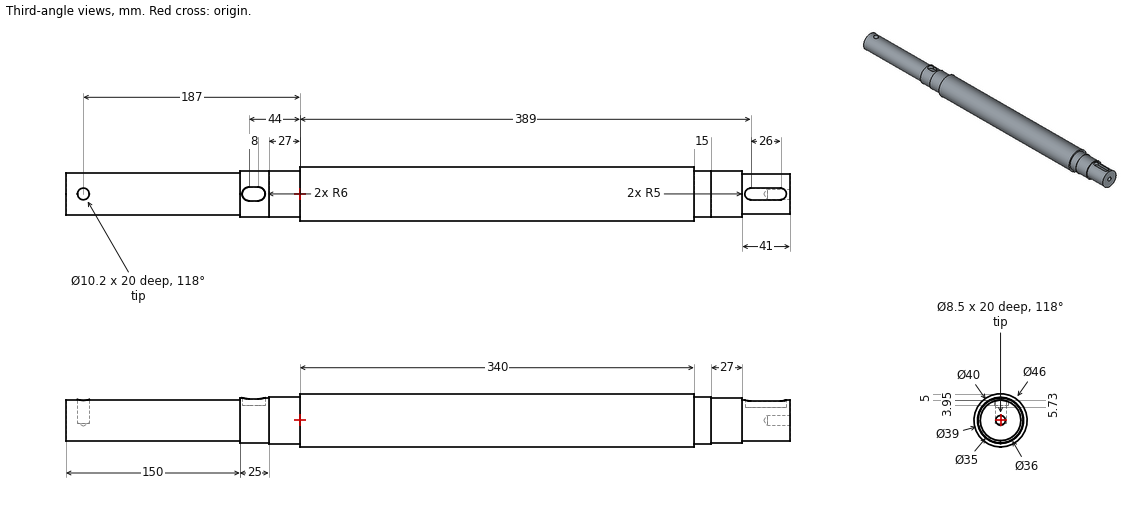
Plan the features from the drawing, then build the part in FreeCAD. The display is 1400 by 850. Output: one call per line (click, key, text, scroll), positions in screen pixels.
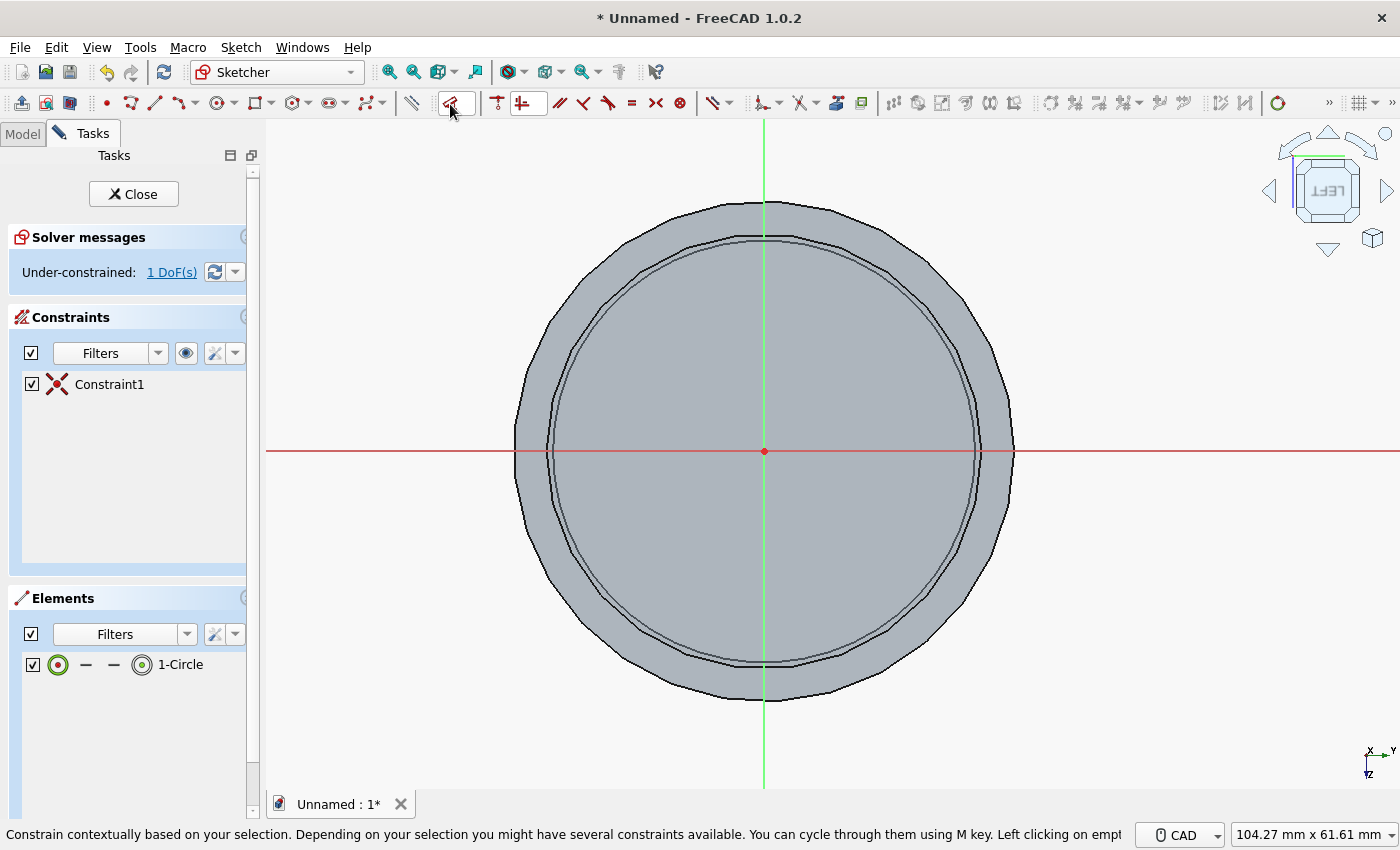
click(913, 302)
click(936, 279)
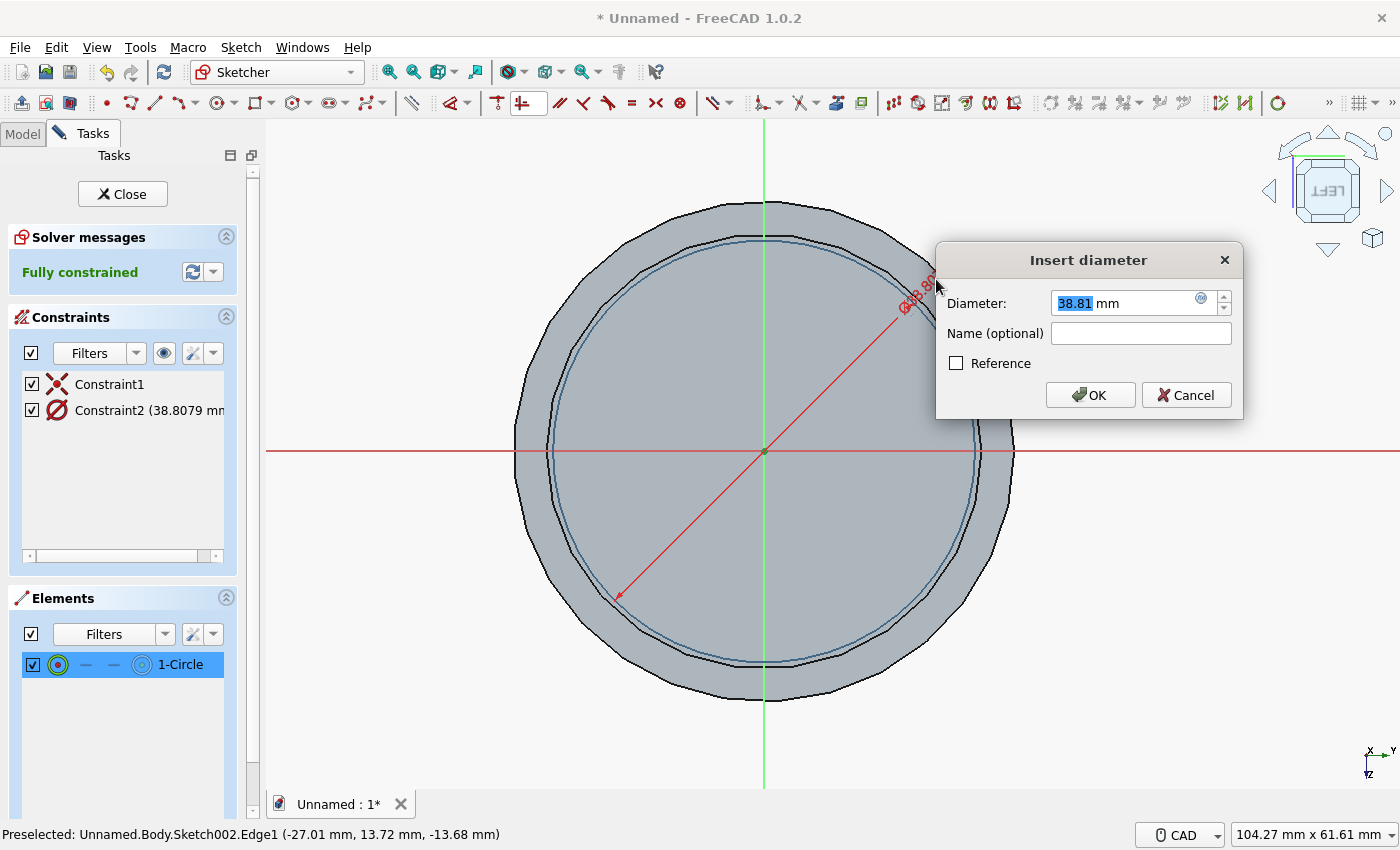
text(39)
key(Return)
key(Escape)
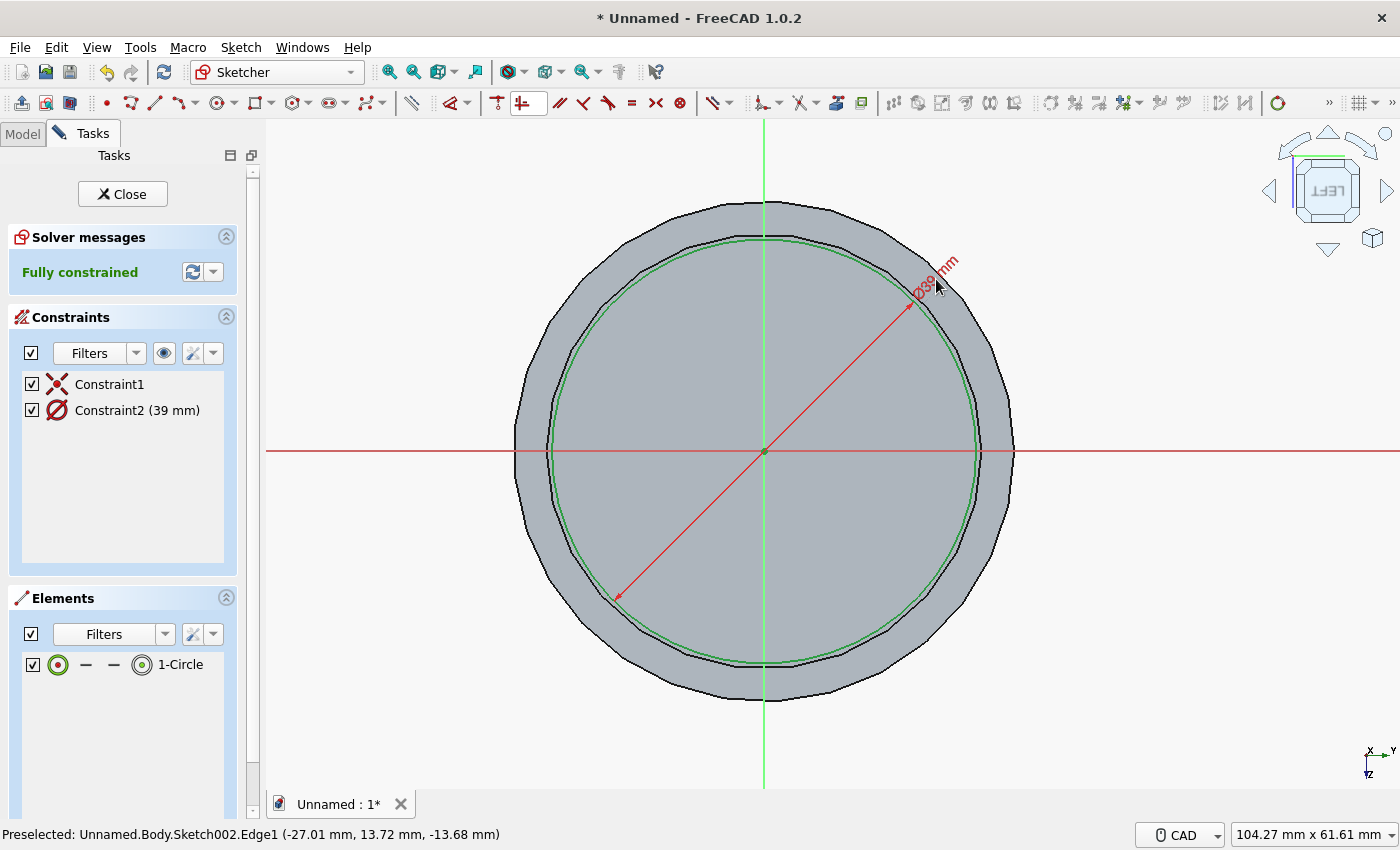
click(123, 194)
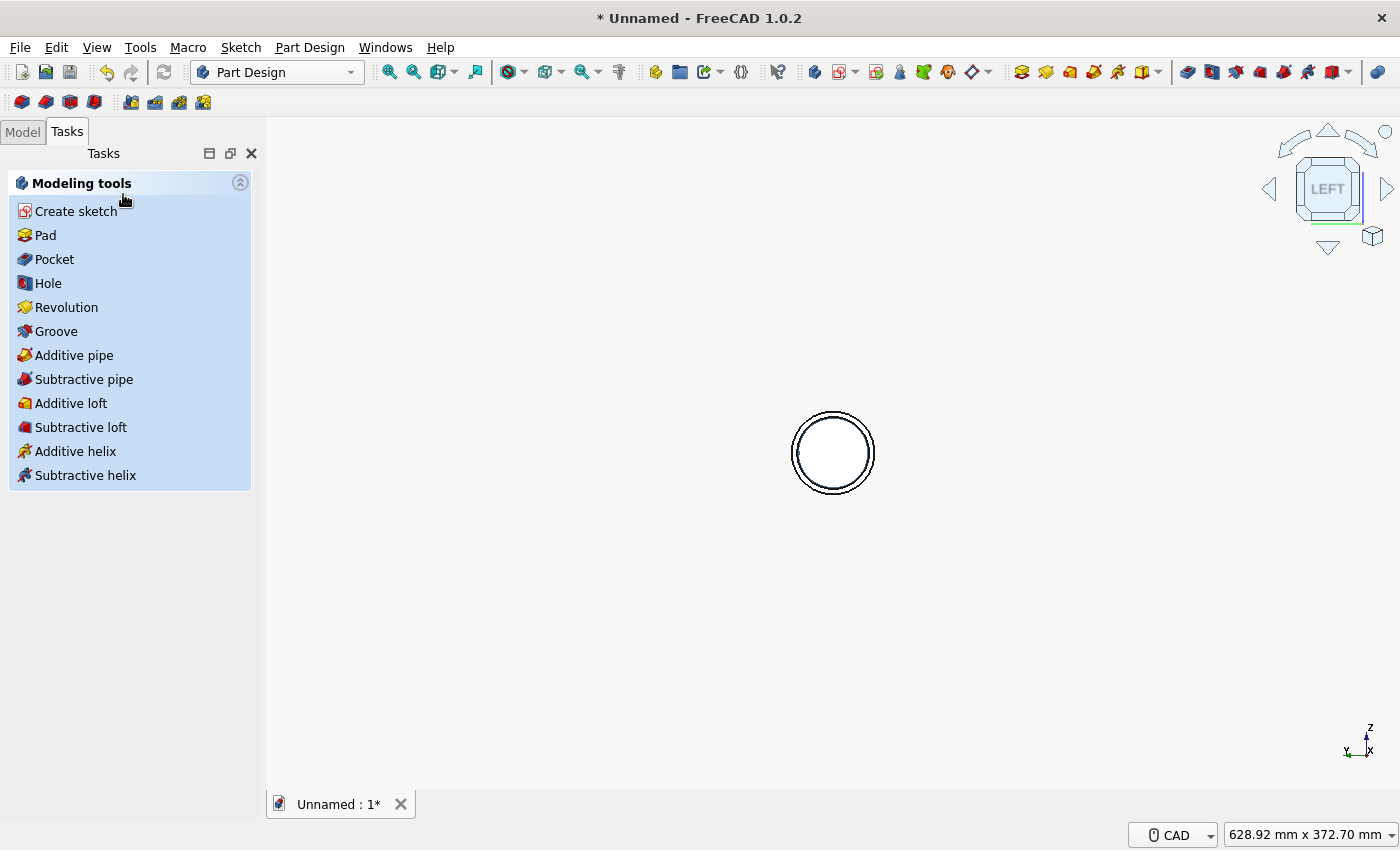
click(1022, 72)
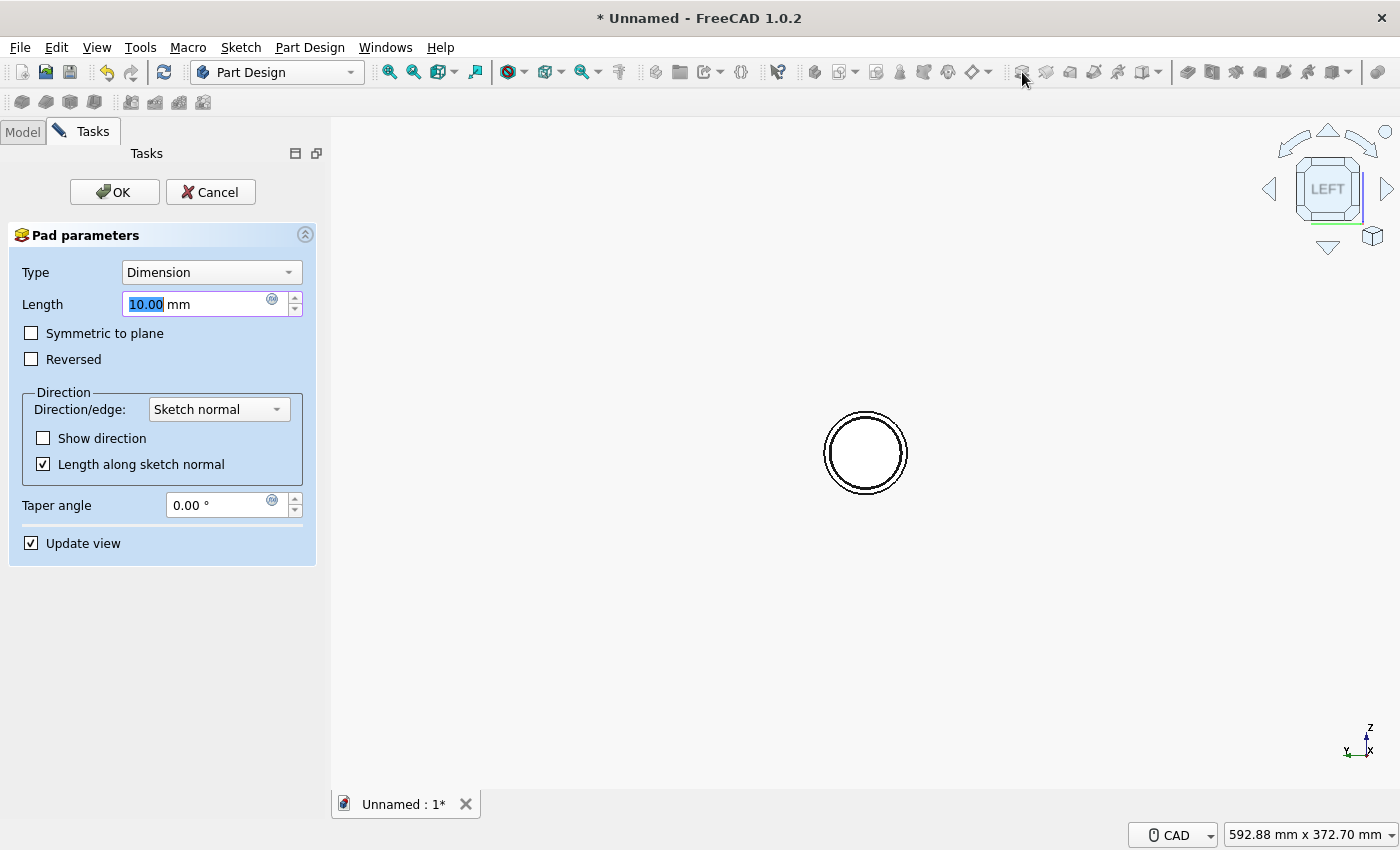
text(25)
key(Tab)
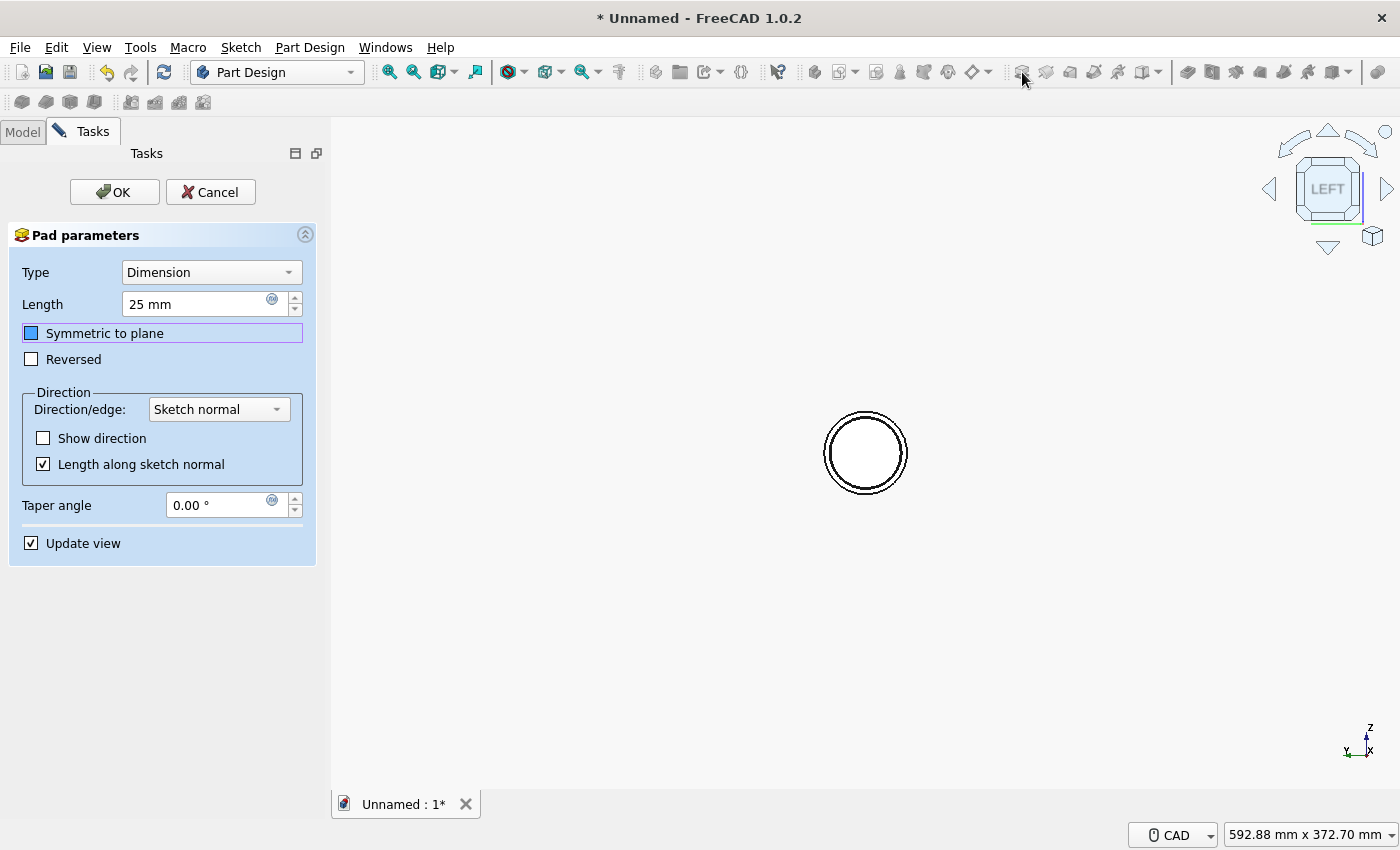
click(115, 192)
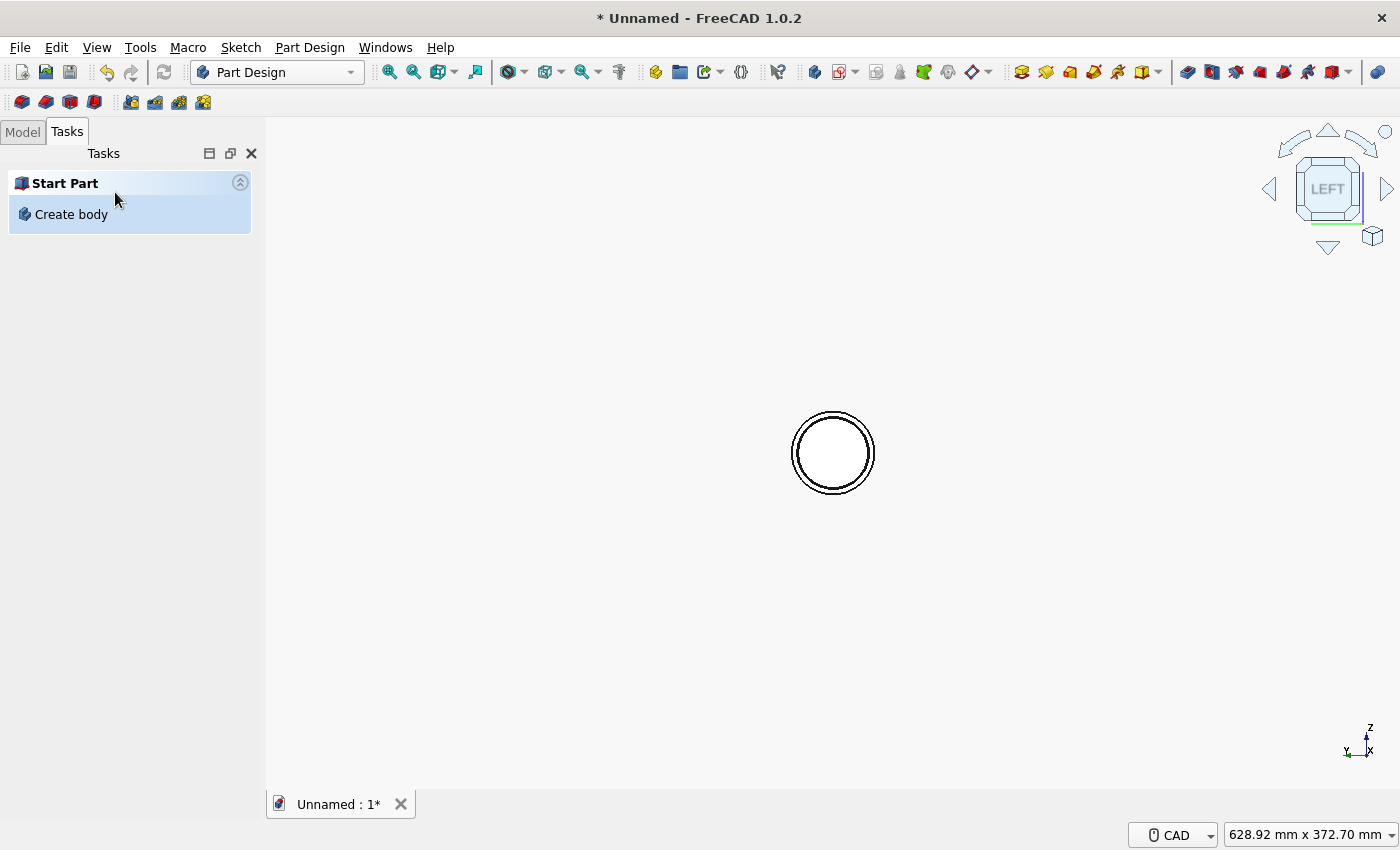
click(390, 72)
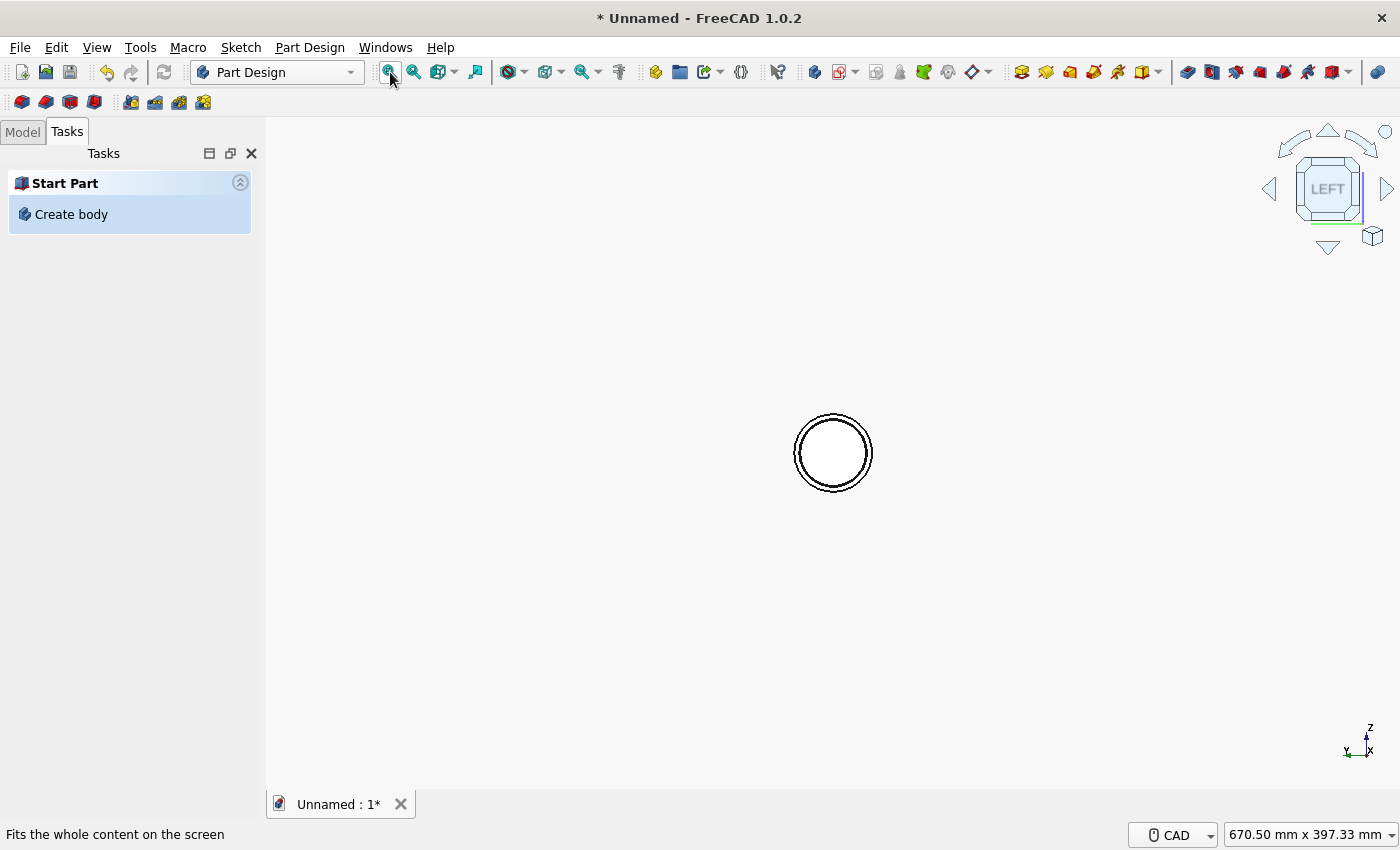
click(23, 131)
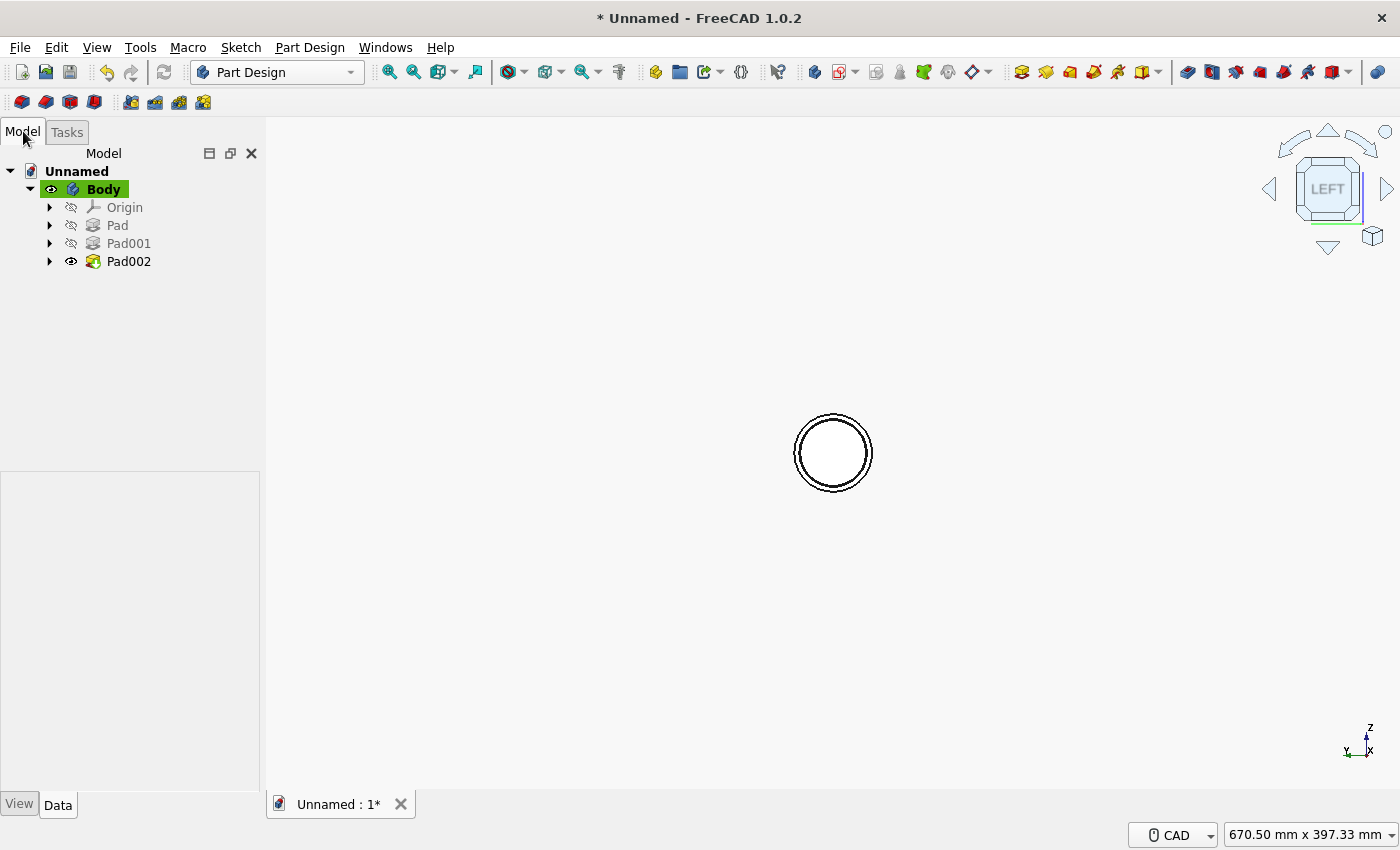
click(50, 207)